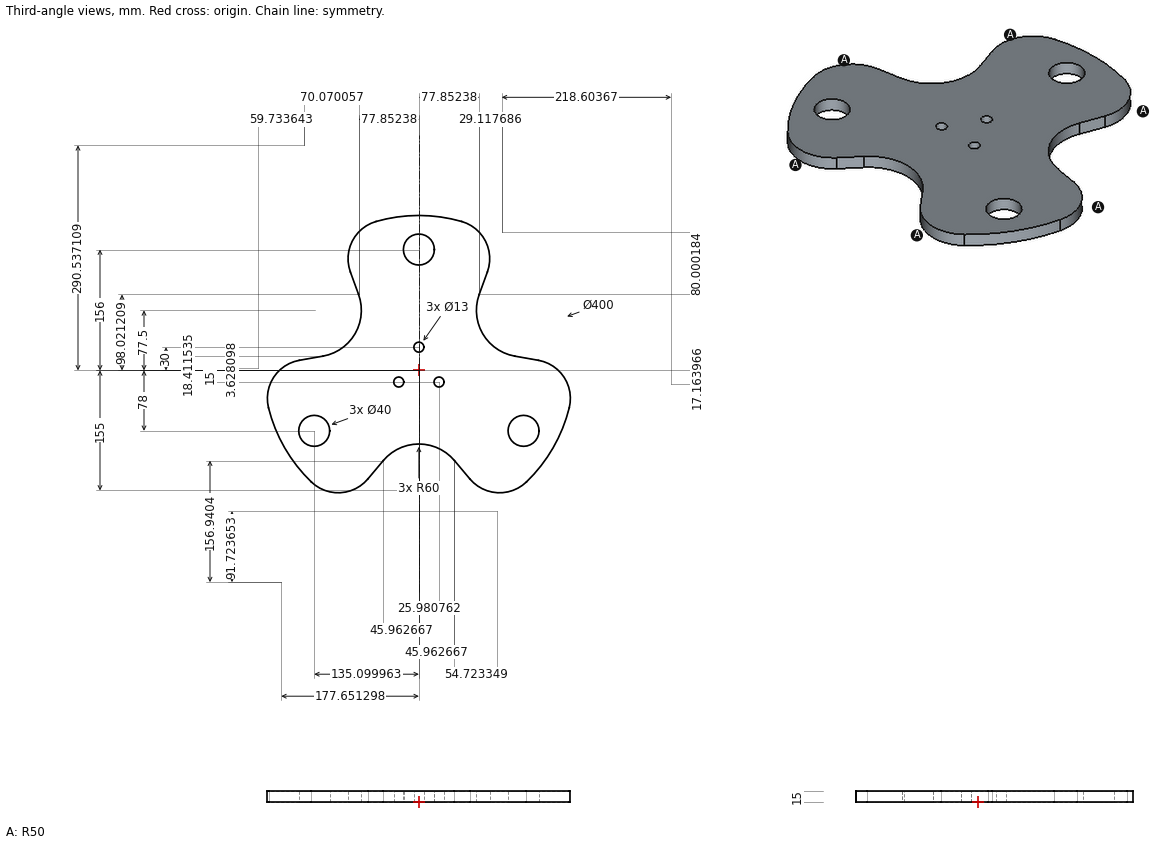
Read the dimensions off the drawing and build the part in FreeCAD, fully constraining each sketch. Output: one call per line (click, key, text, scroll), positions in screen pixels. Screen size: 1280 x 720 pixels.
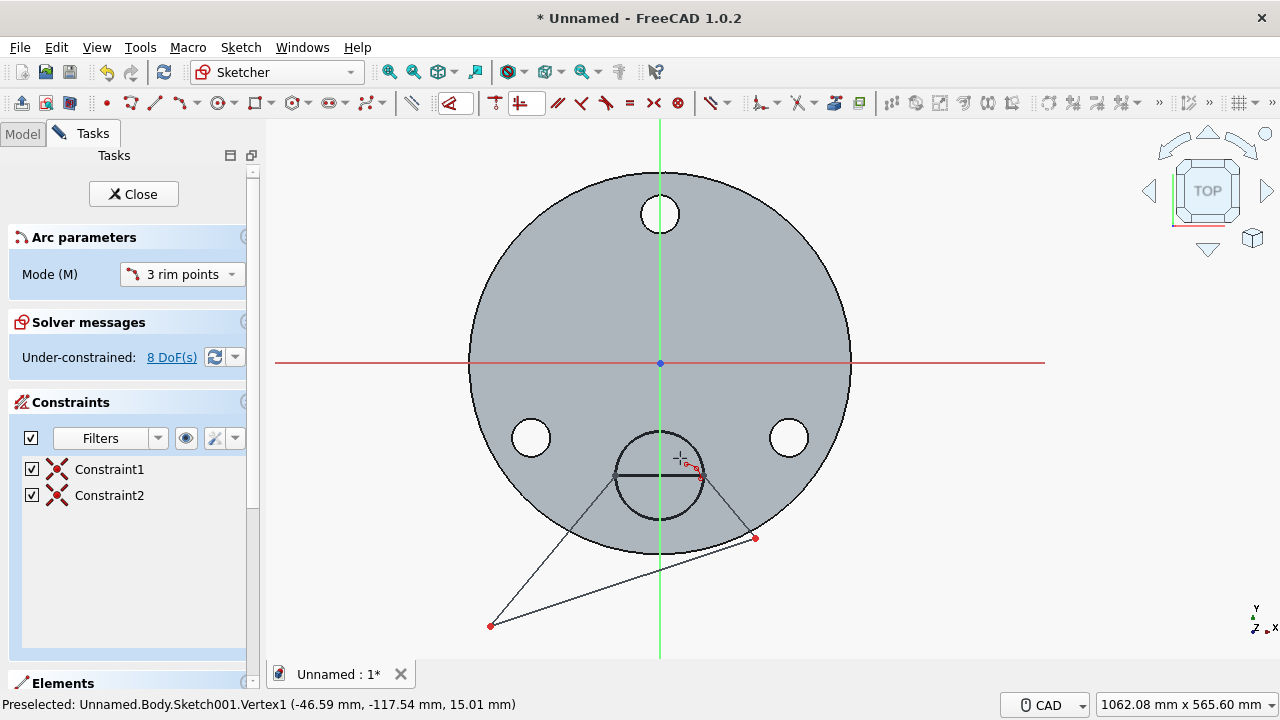
click(680, 458)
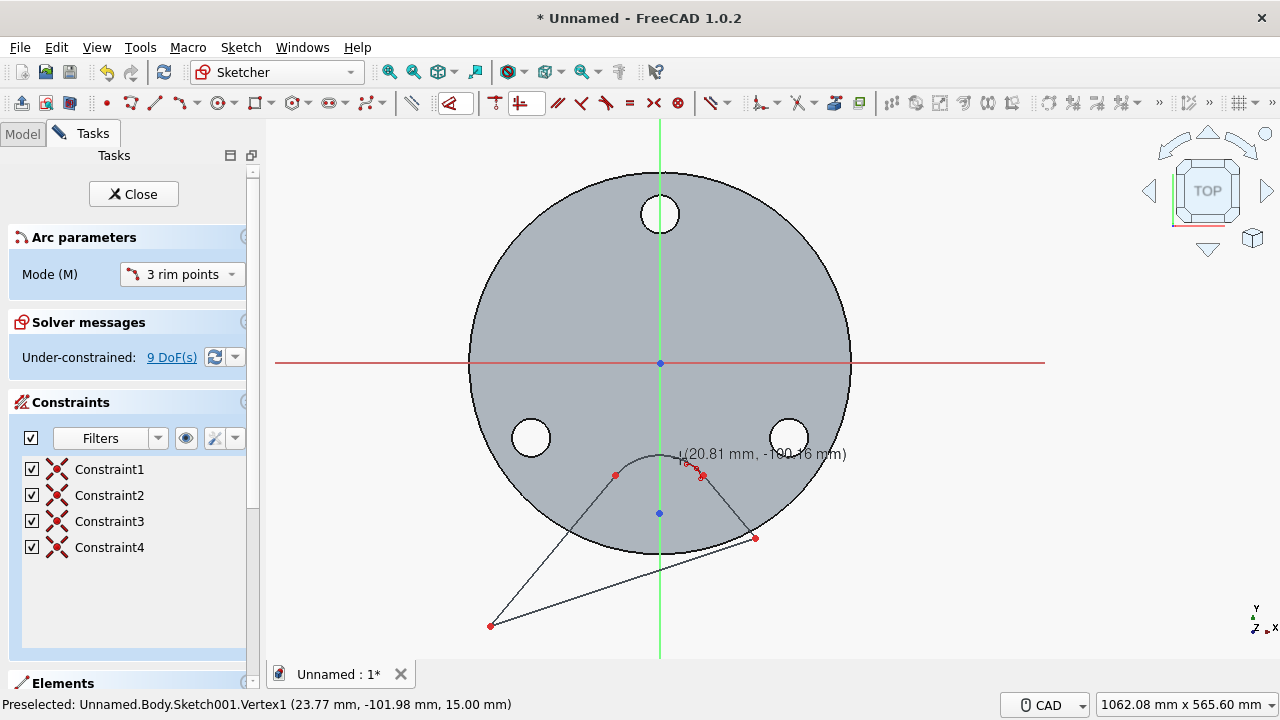
click(132, 104)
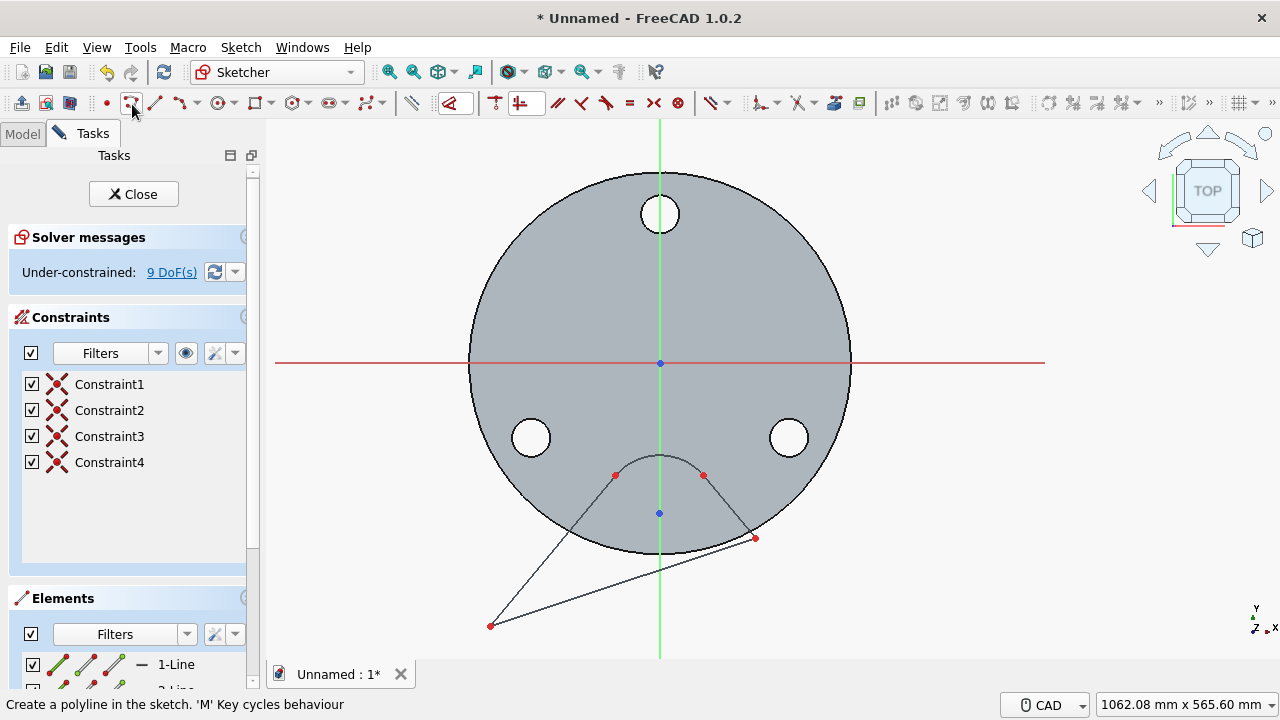
click(586, 270)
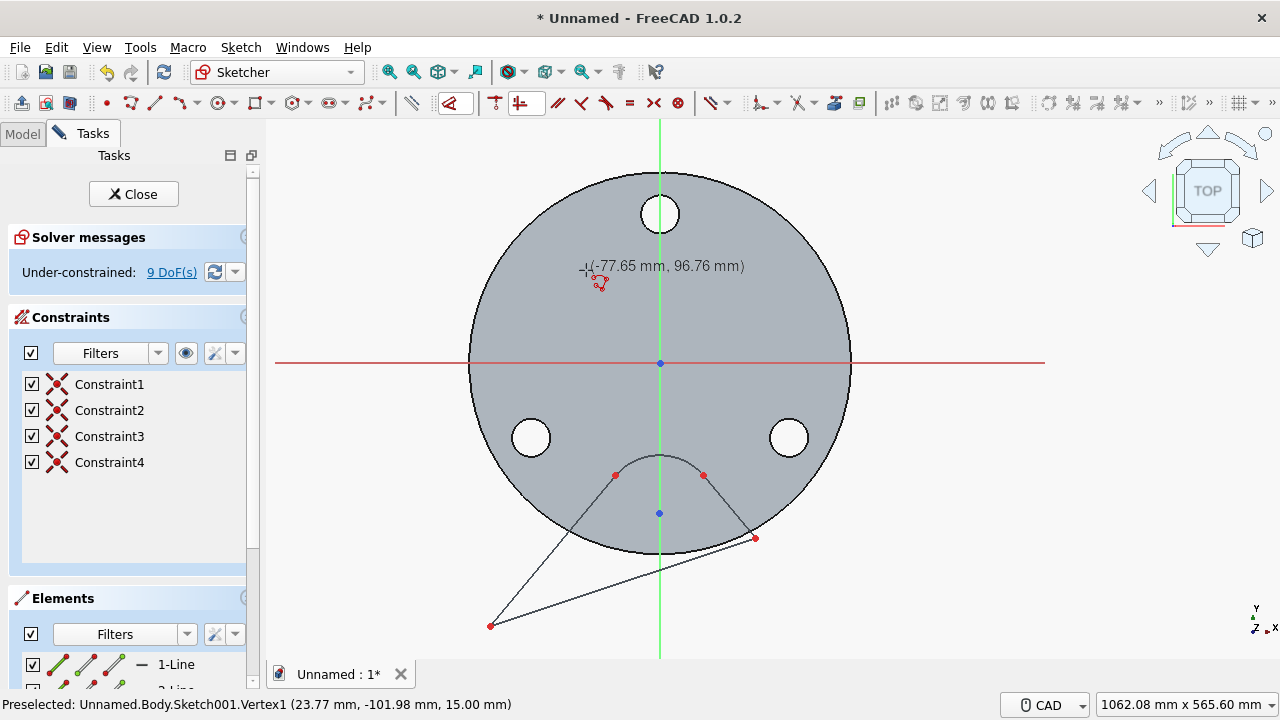
scroll(680, 458, down, 2)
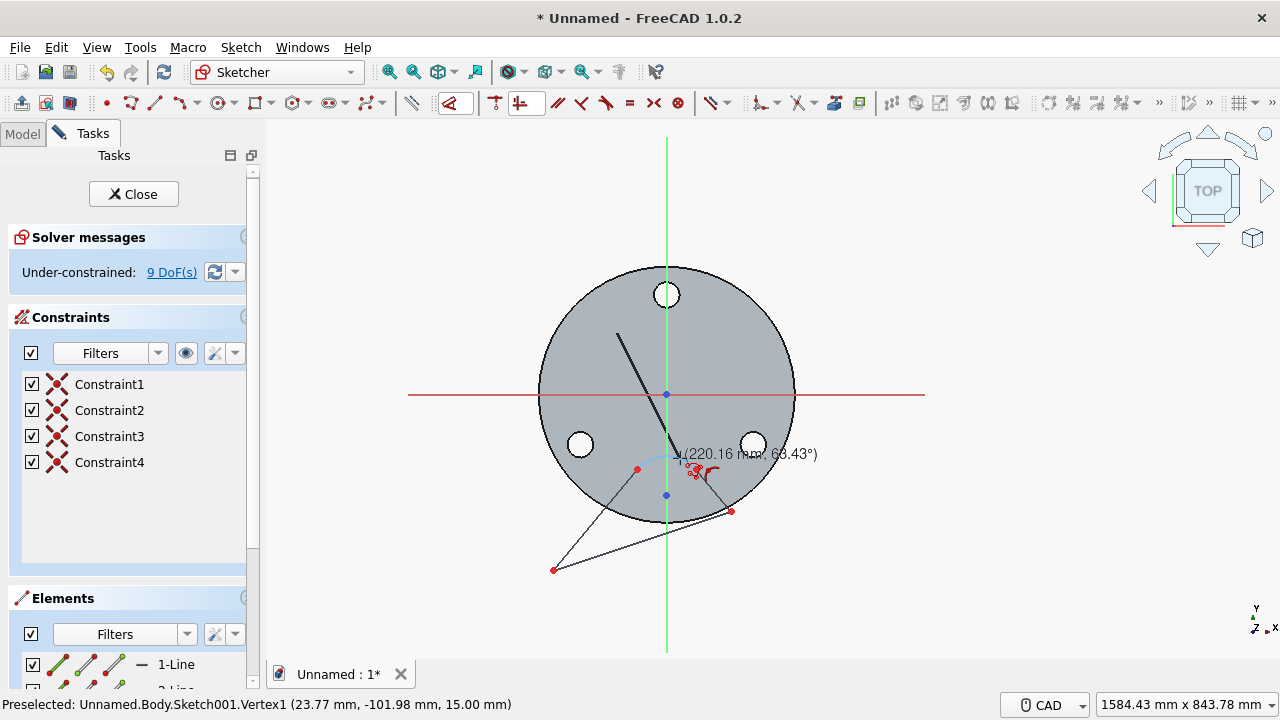
click(572, 209)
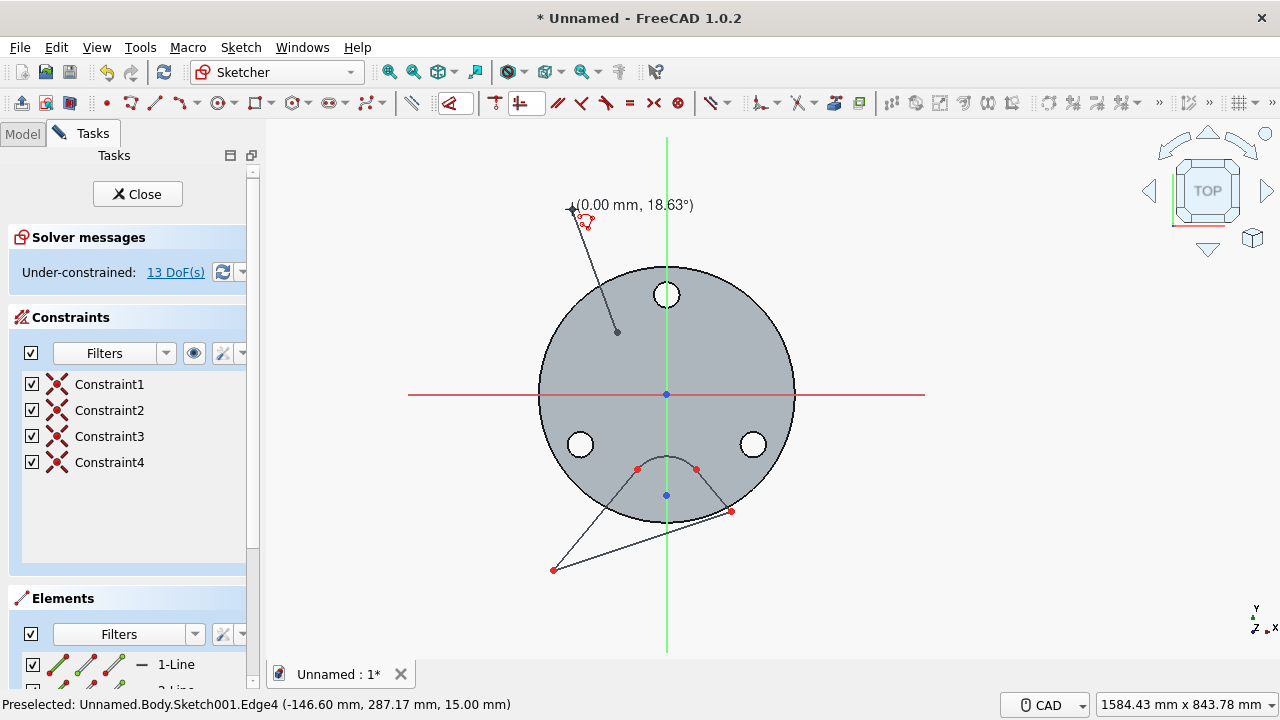
scroll(534, 392, up, 10)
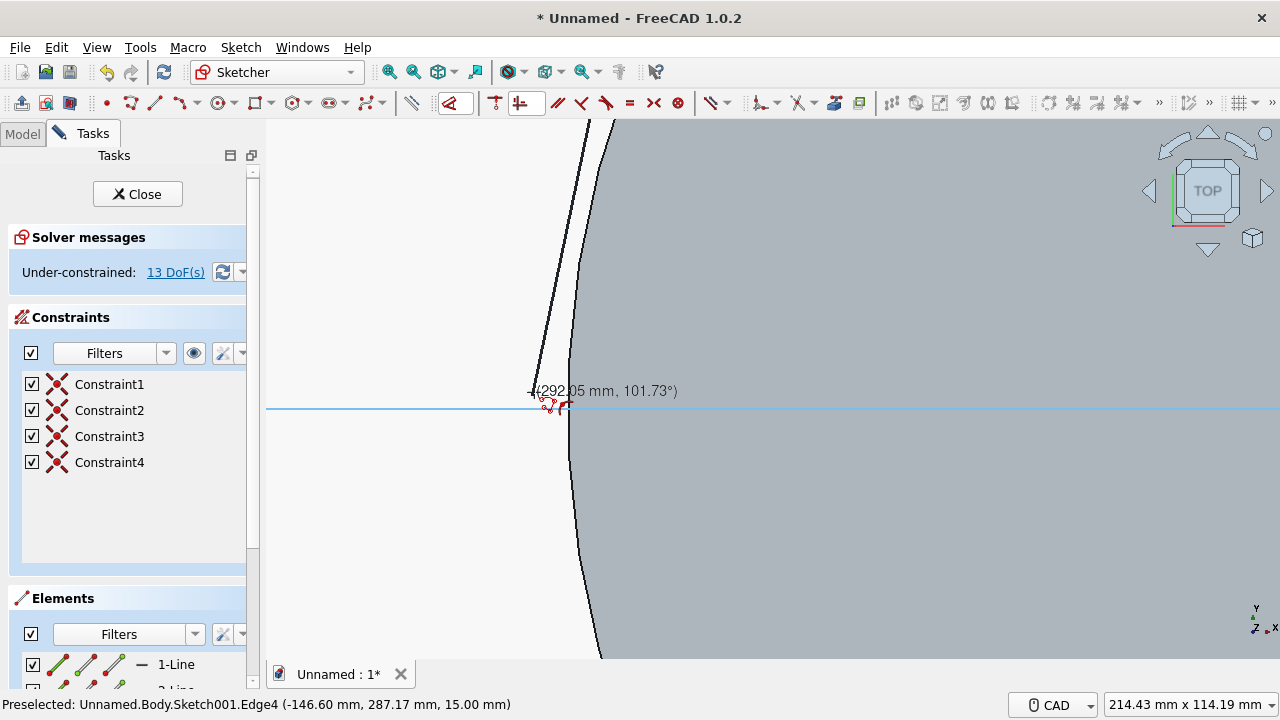
click(532, 392)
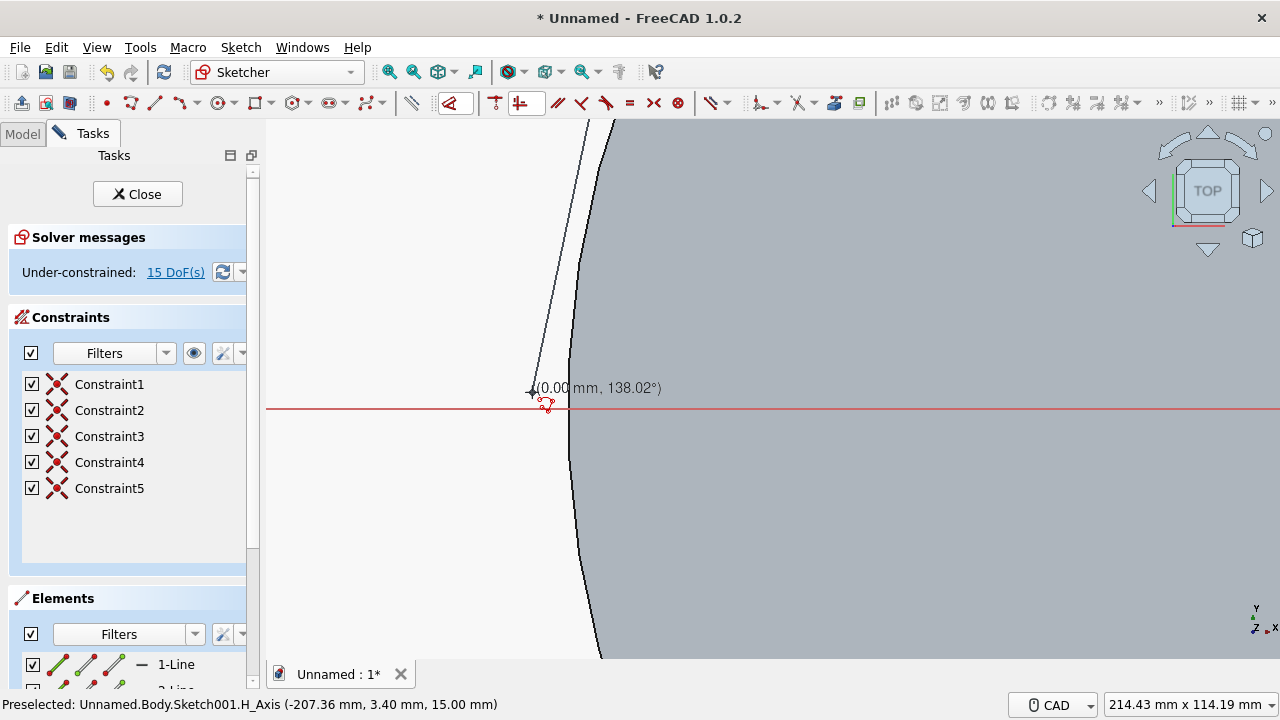
scroll(534, 392, down, 10)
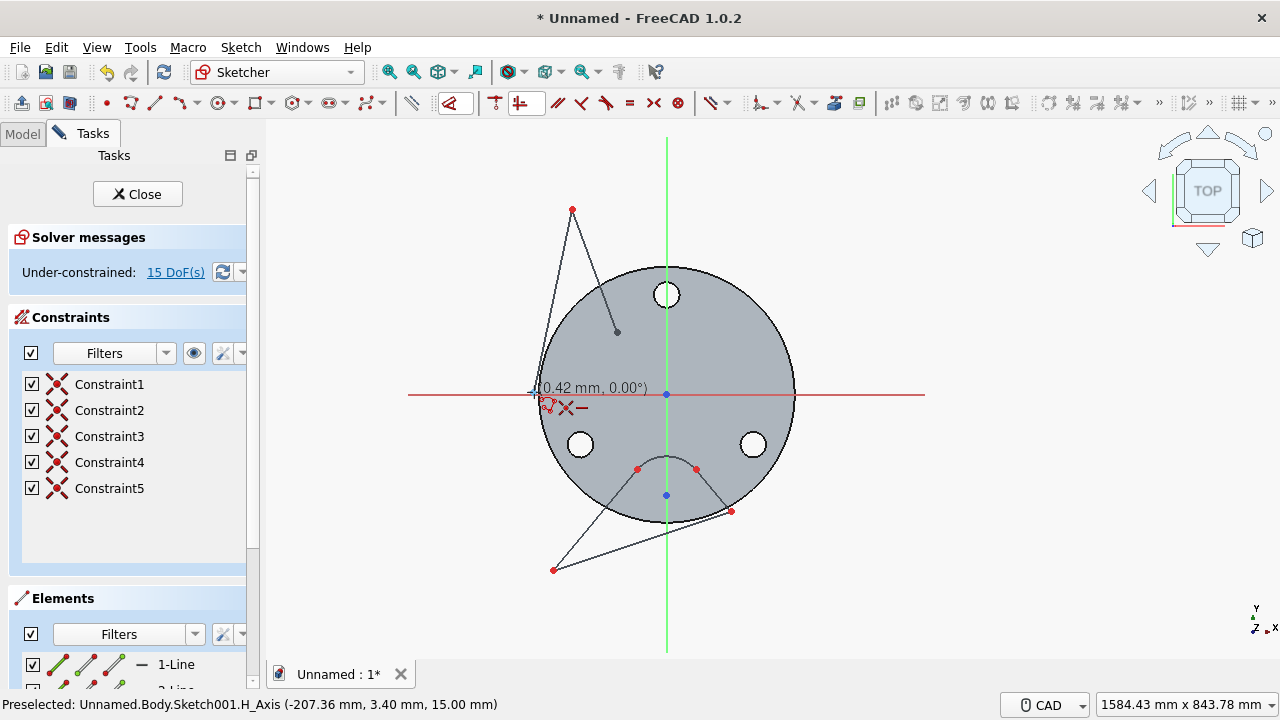
scroll(588, 383, up, 2)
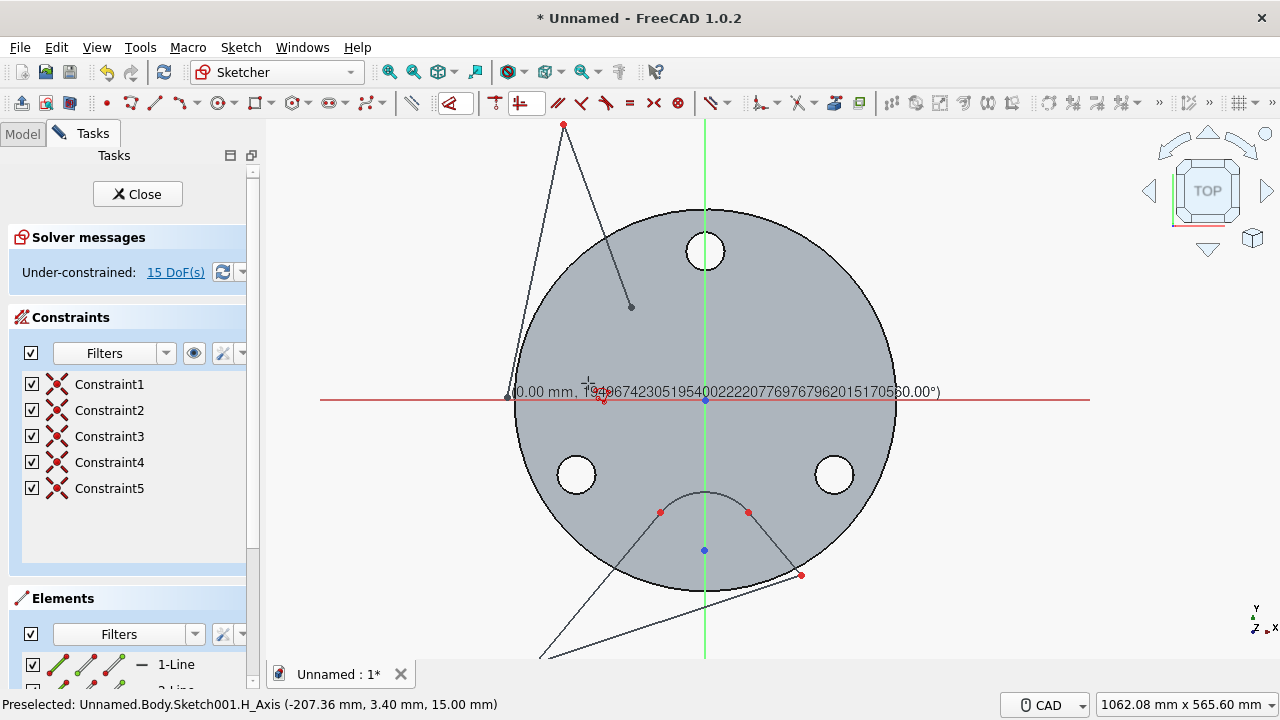
click(587, 383)
right_click(587, 383)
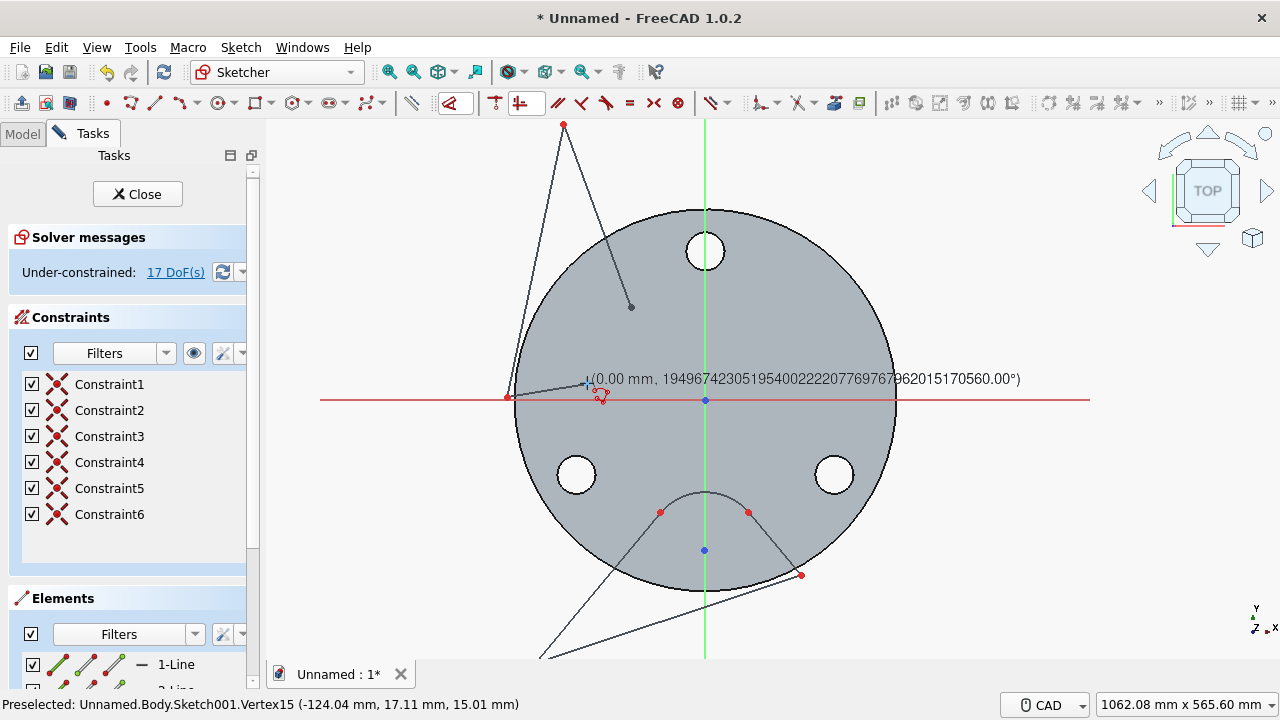
click(180, 104)